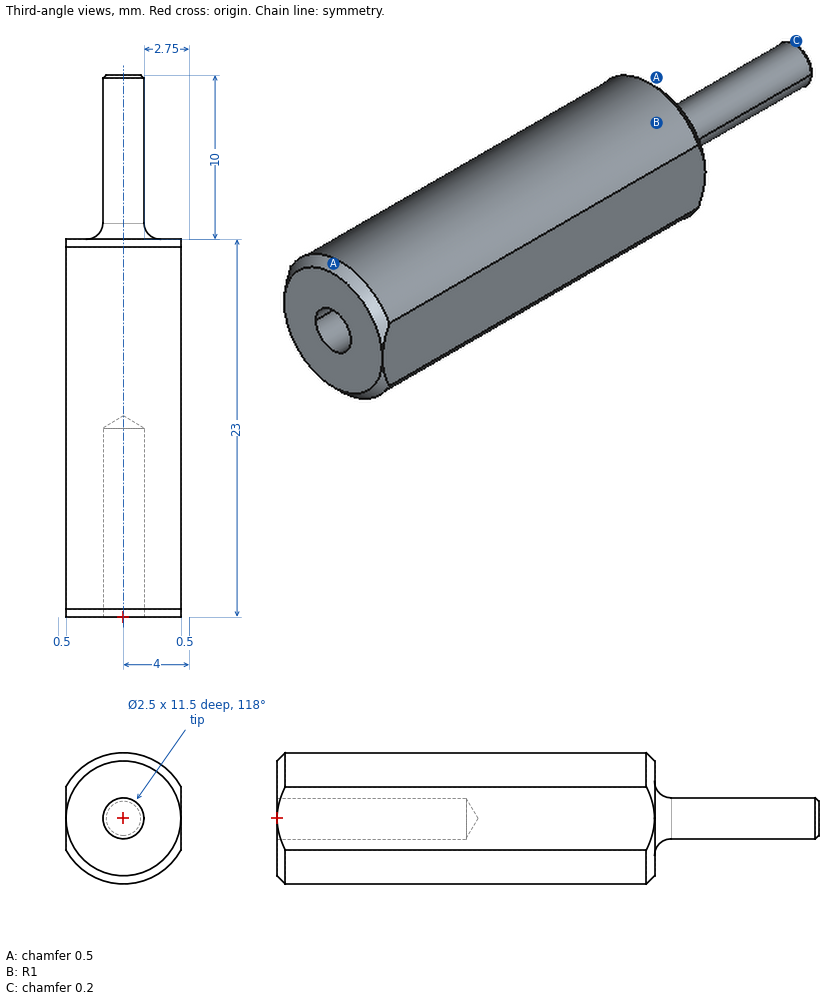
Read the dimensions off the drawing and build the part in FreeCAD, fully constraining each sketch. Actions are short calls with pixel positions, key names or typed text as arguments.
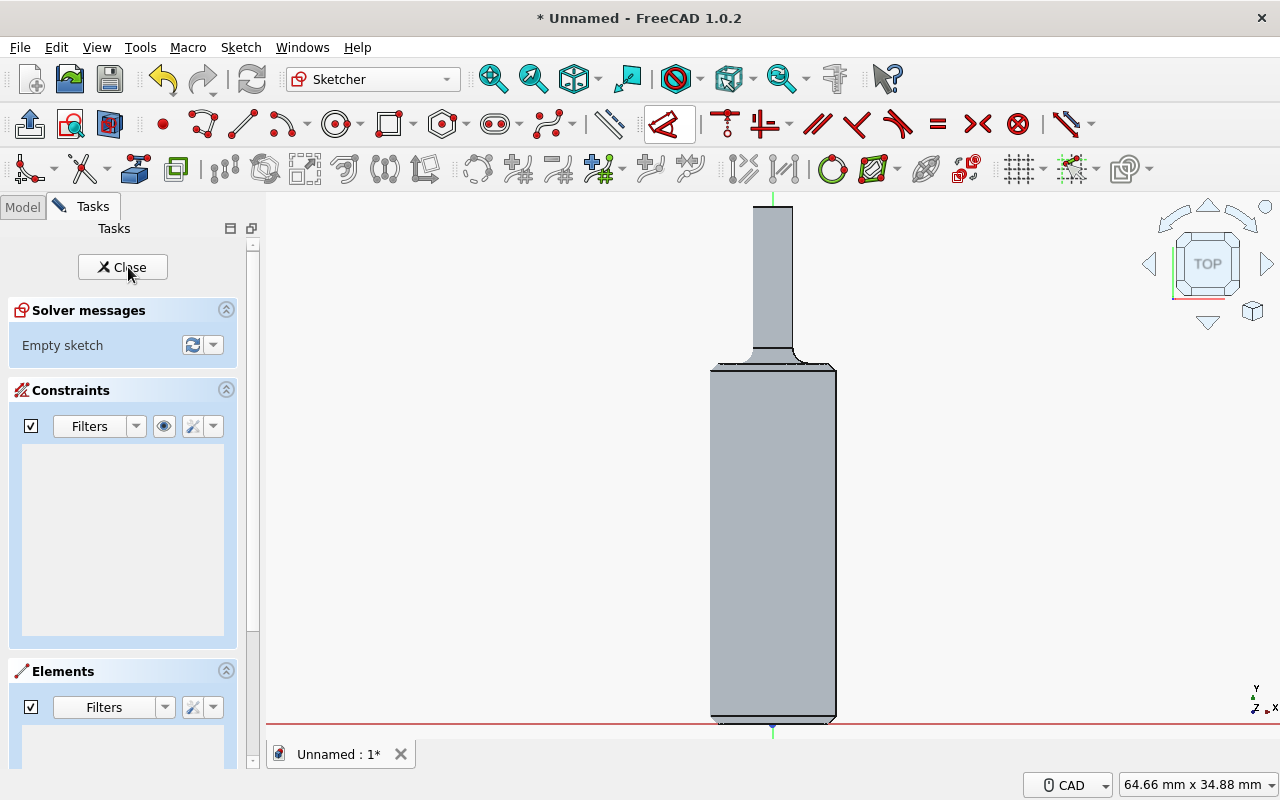
key(q)
key(s)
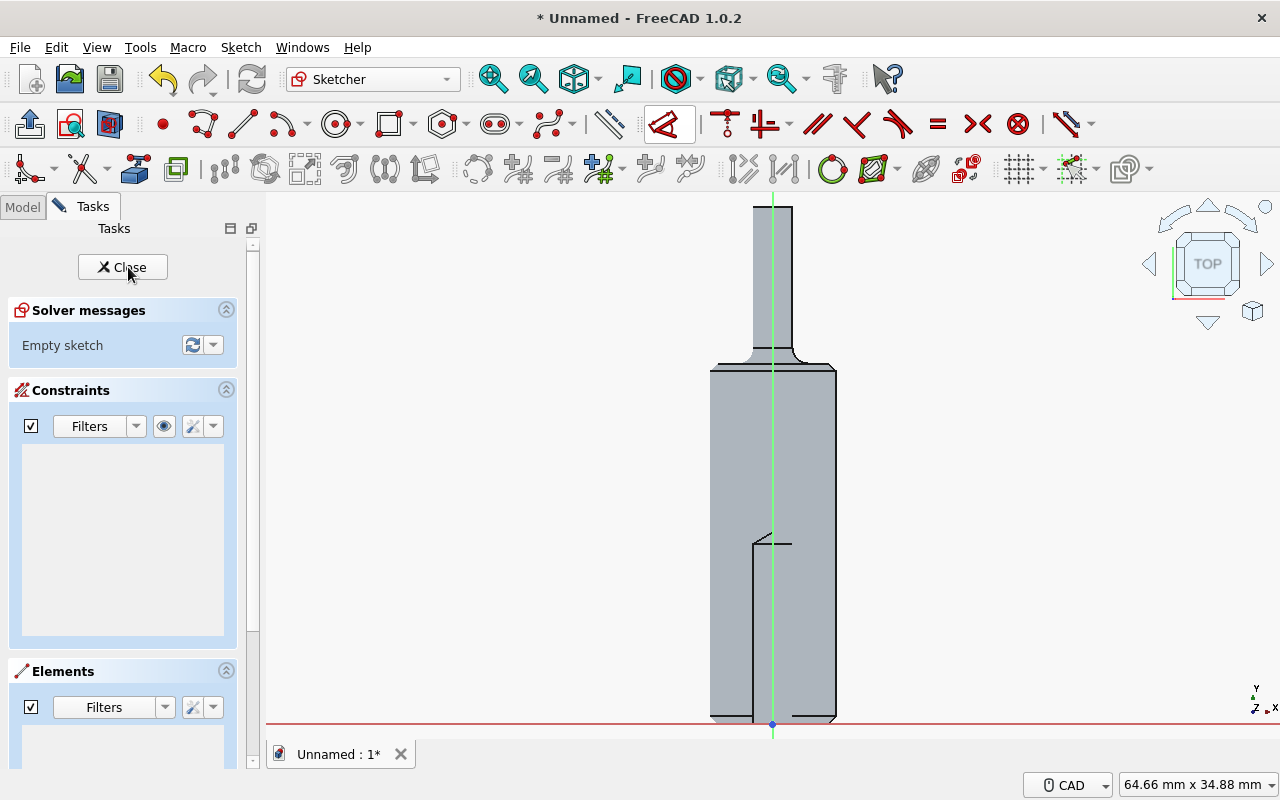
scroll(396, 220, down, 1)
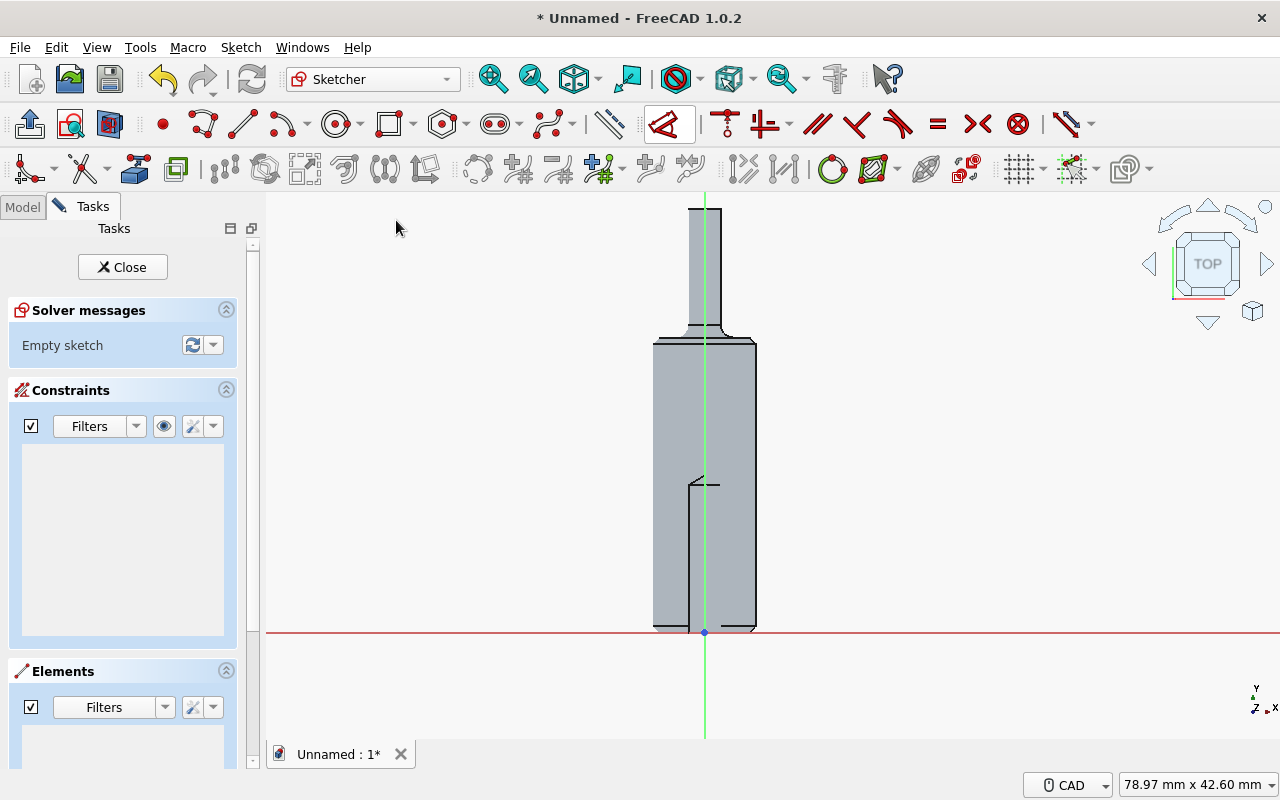
key(g)
key(r)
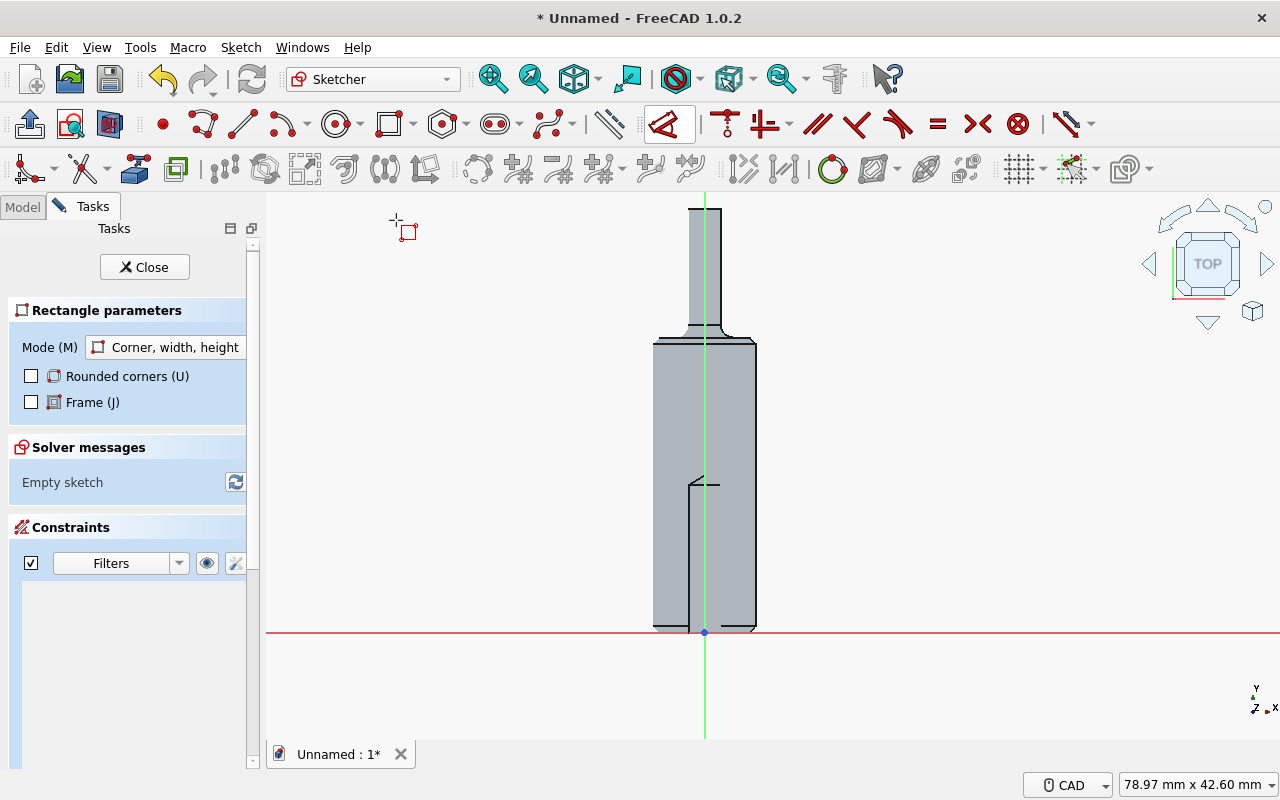
scroll(750, 338, up, 5)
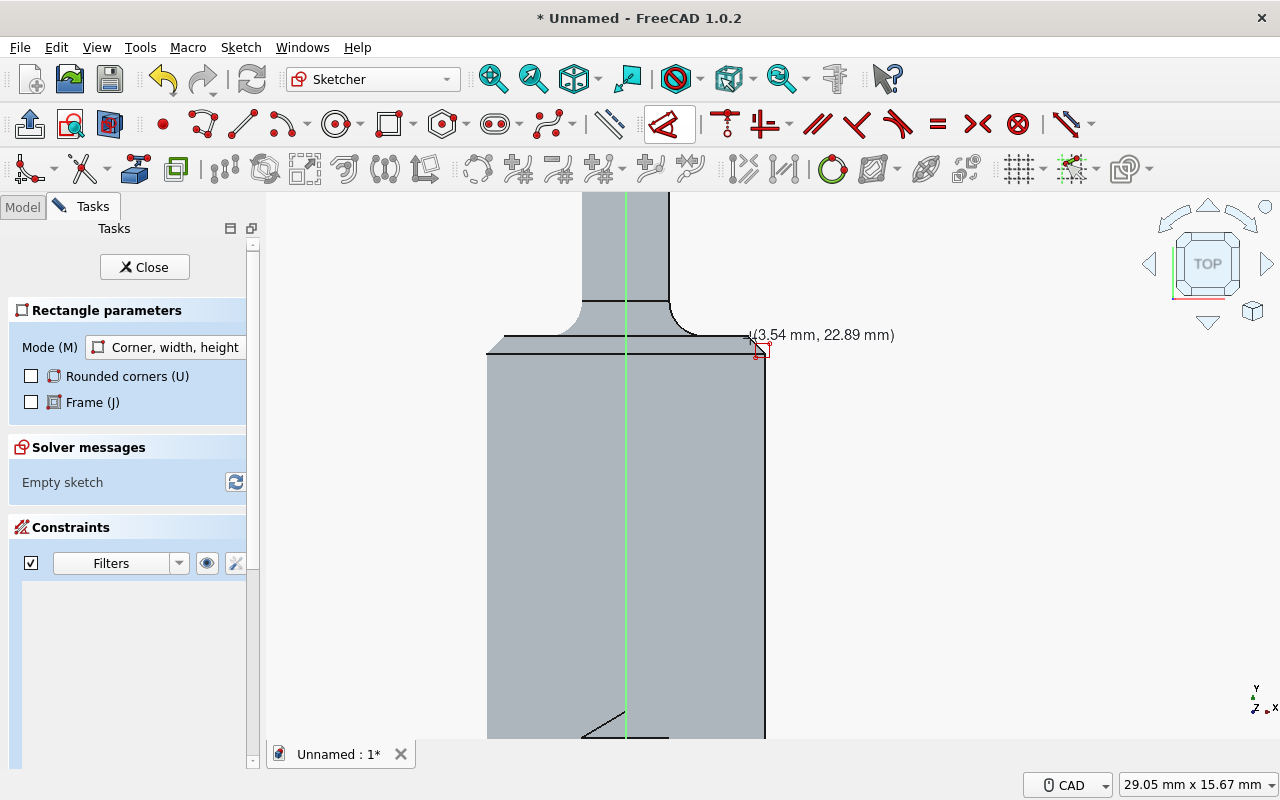
click(748, 336)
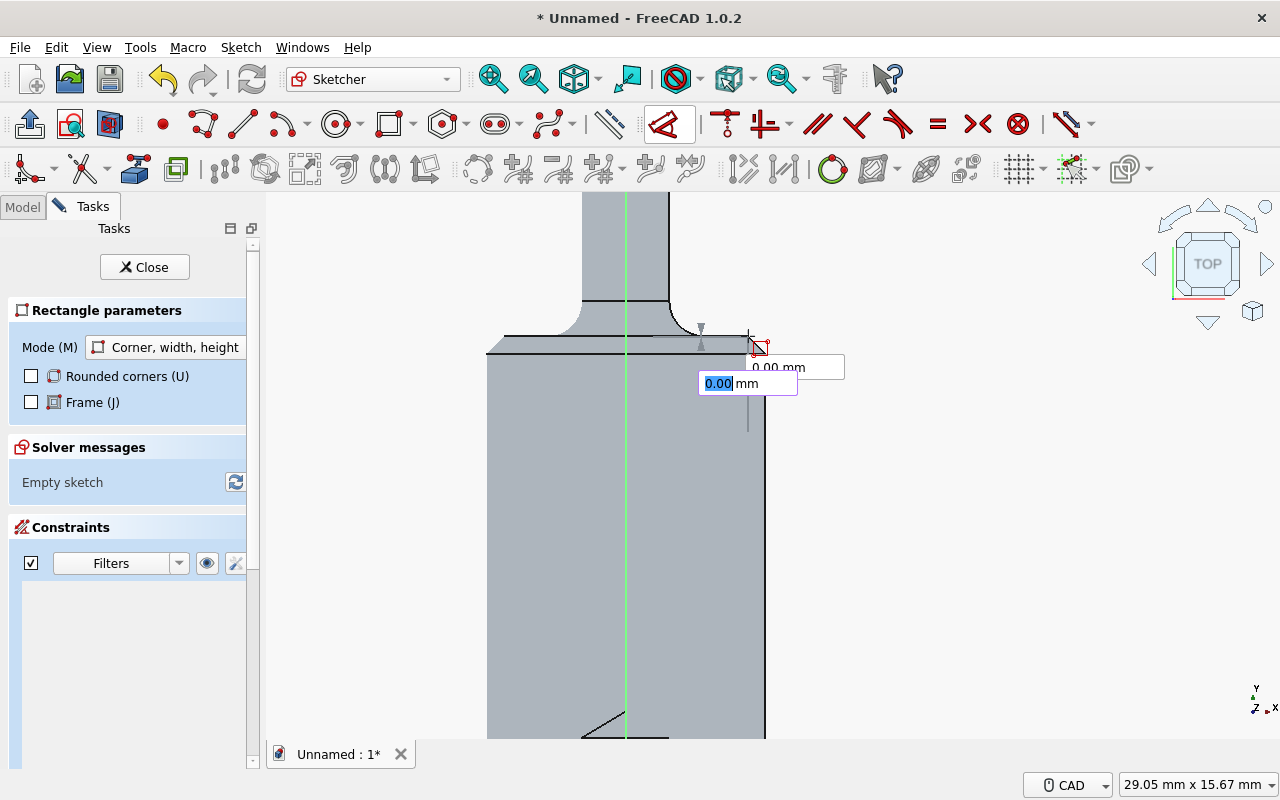
scroll(769, 243, down, 4)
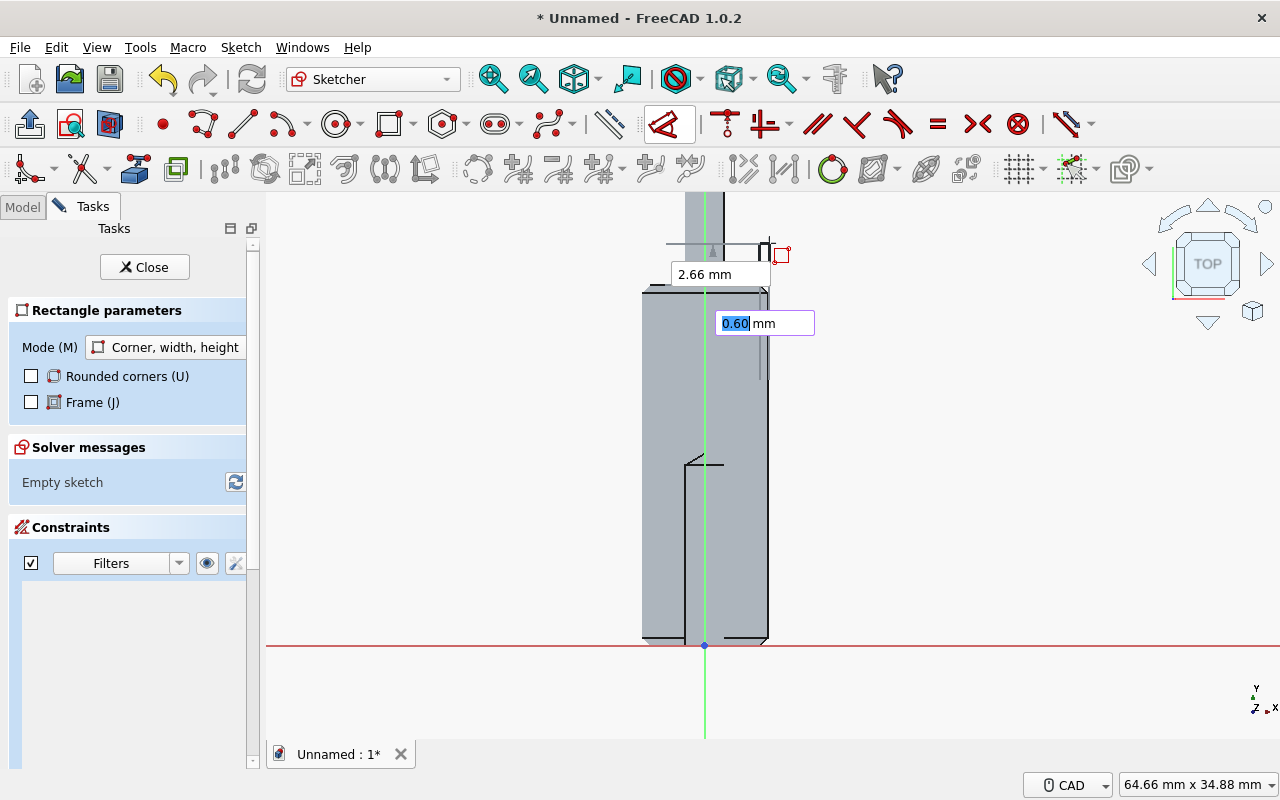
click(768, 646)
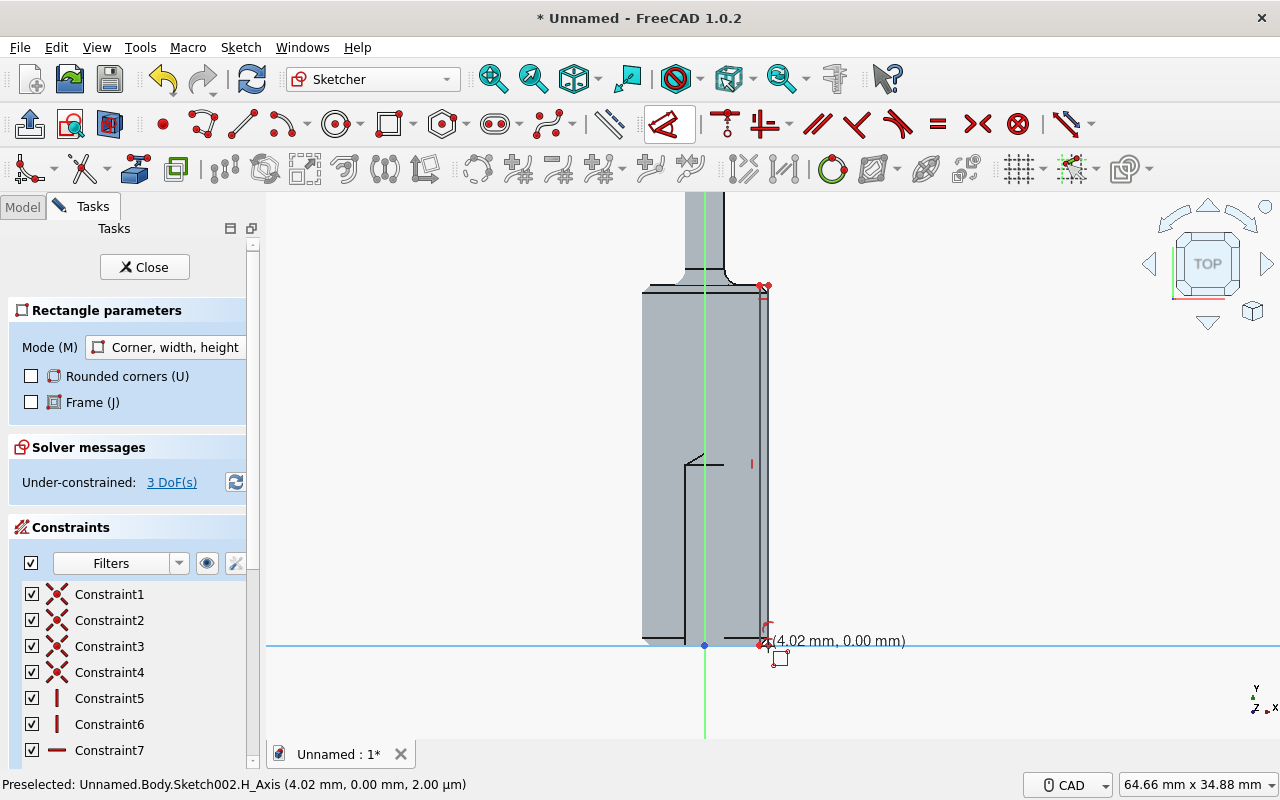
scroll(642, 285, up, 4)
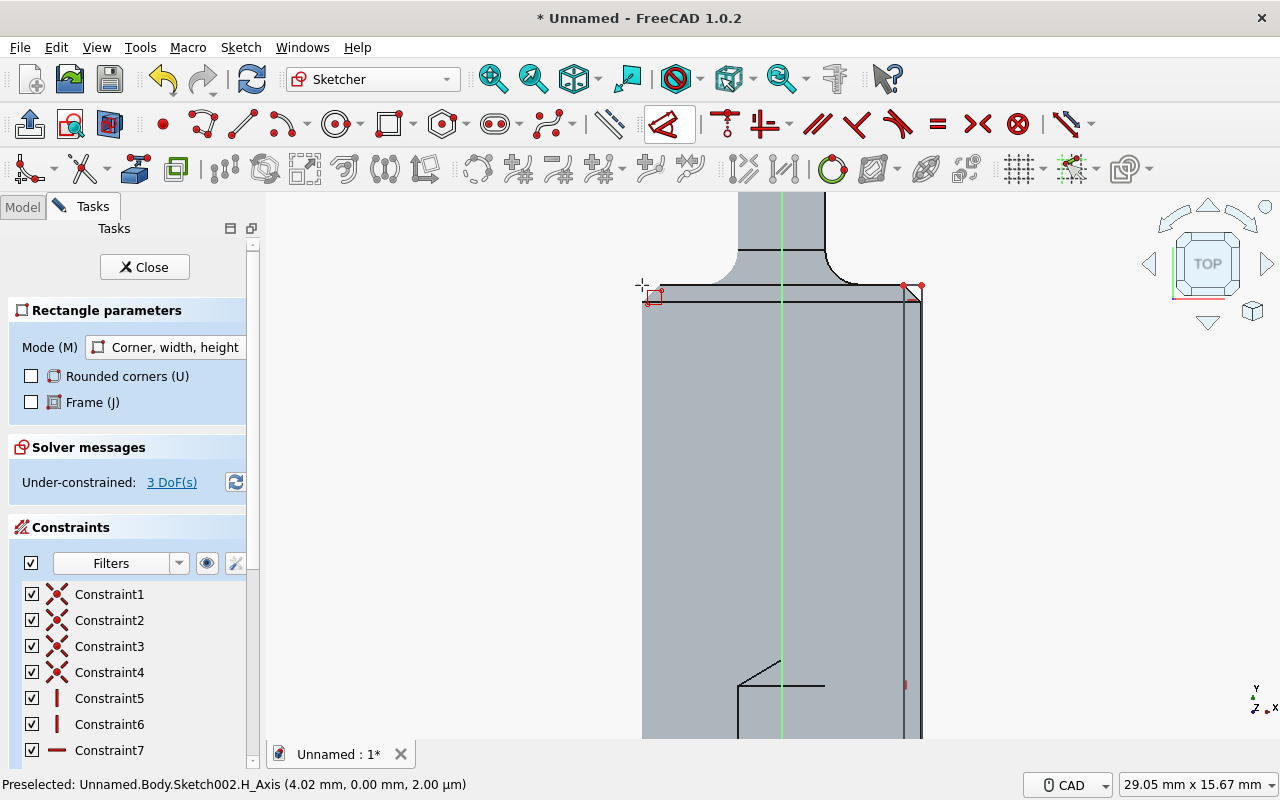
click(642, 285)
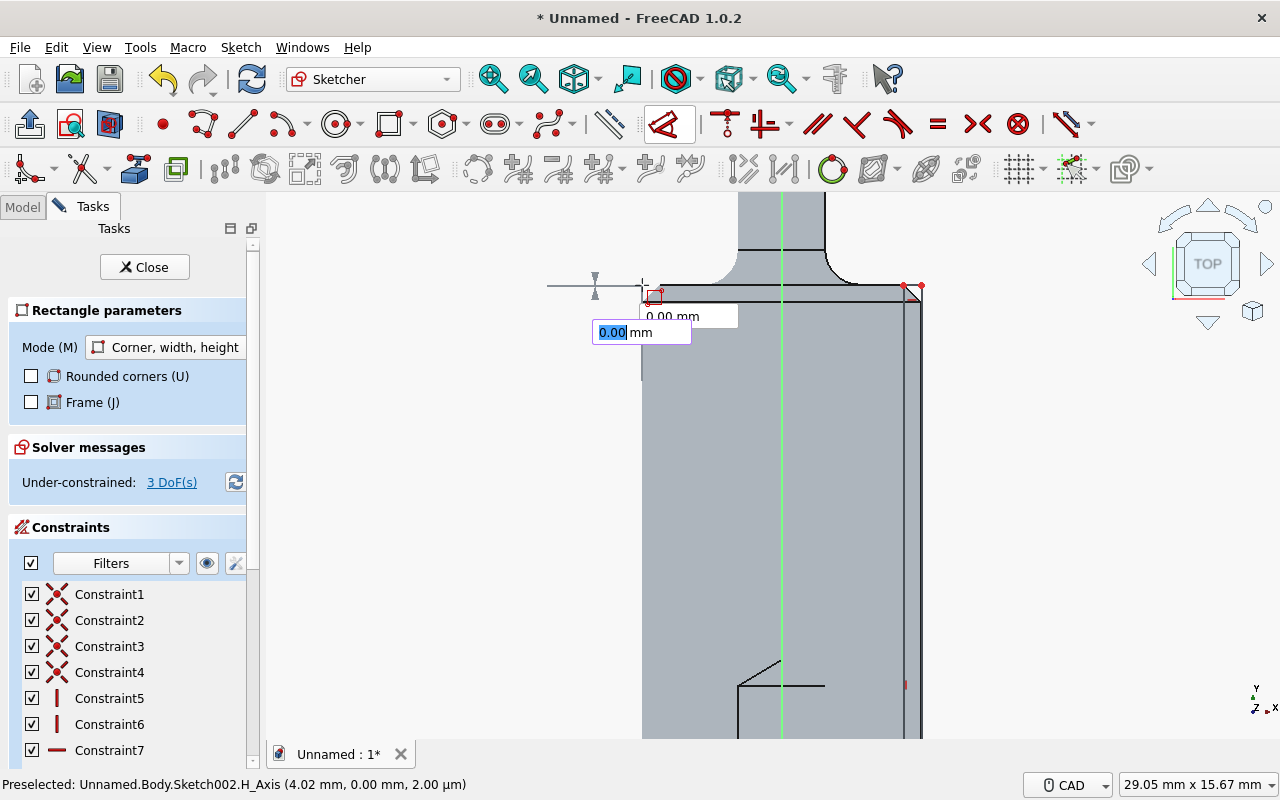
scroll(642, 285, down, 4)